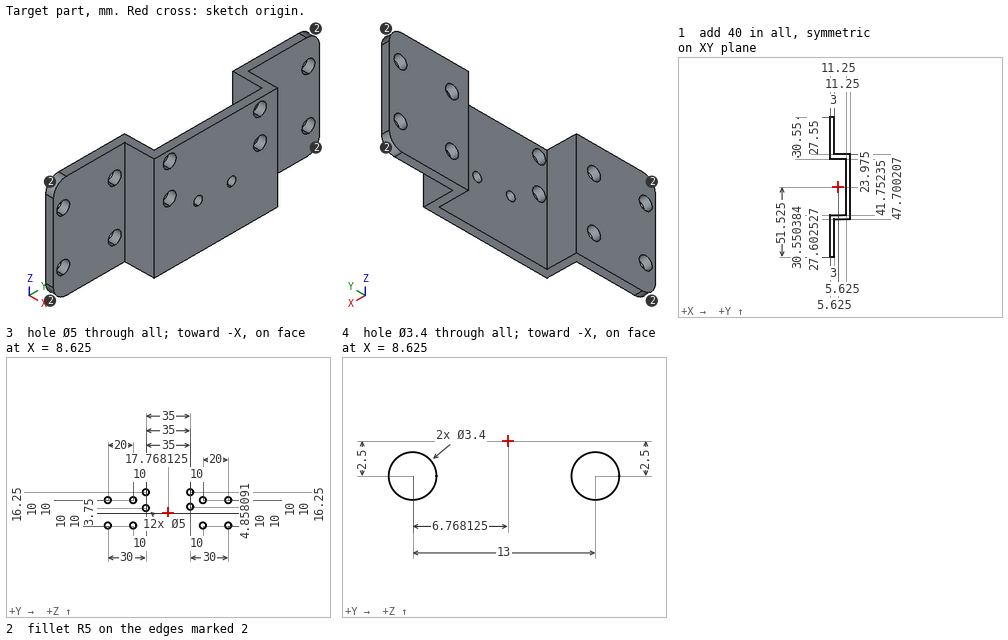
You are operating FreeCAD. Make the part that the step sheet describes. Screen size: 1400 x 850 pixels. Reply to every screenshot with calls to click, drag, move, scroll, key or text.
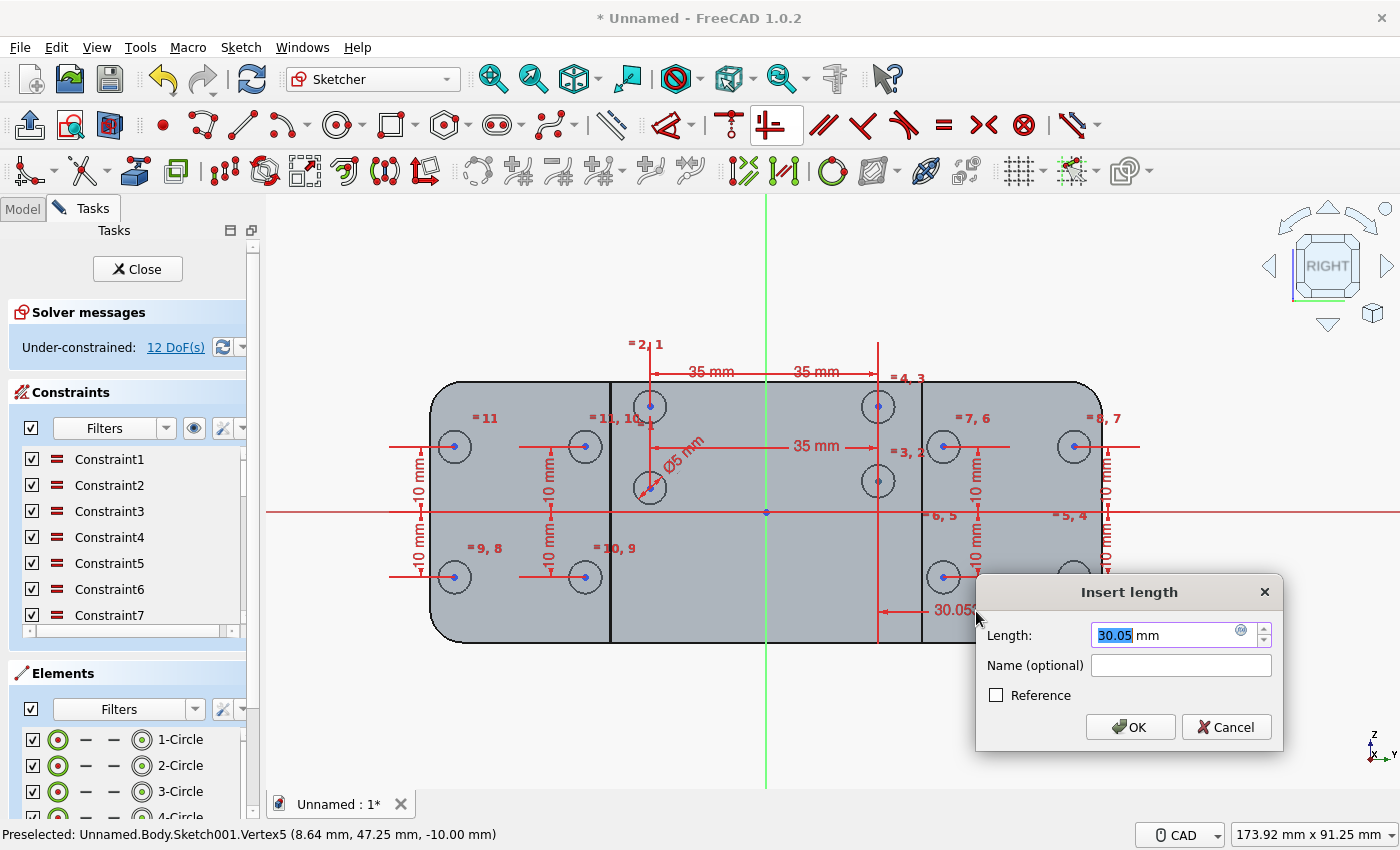
text(30)
key(Return)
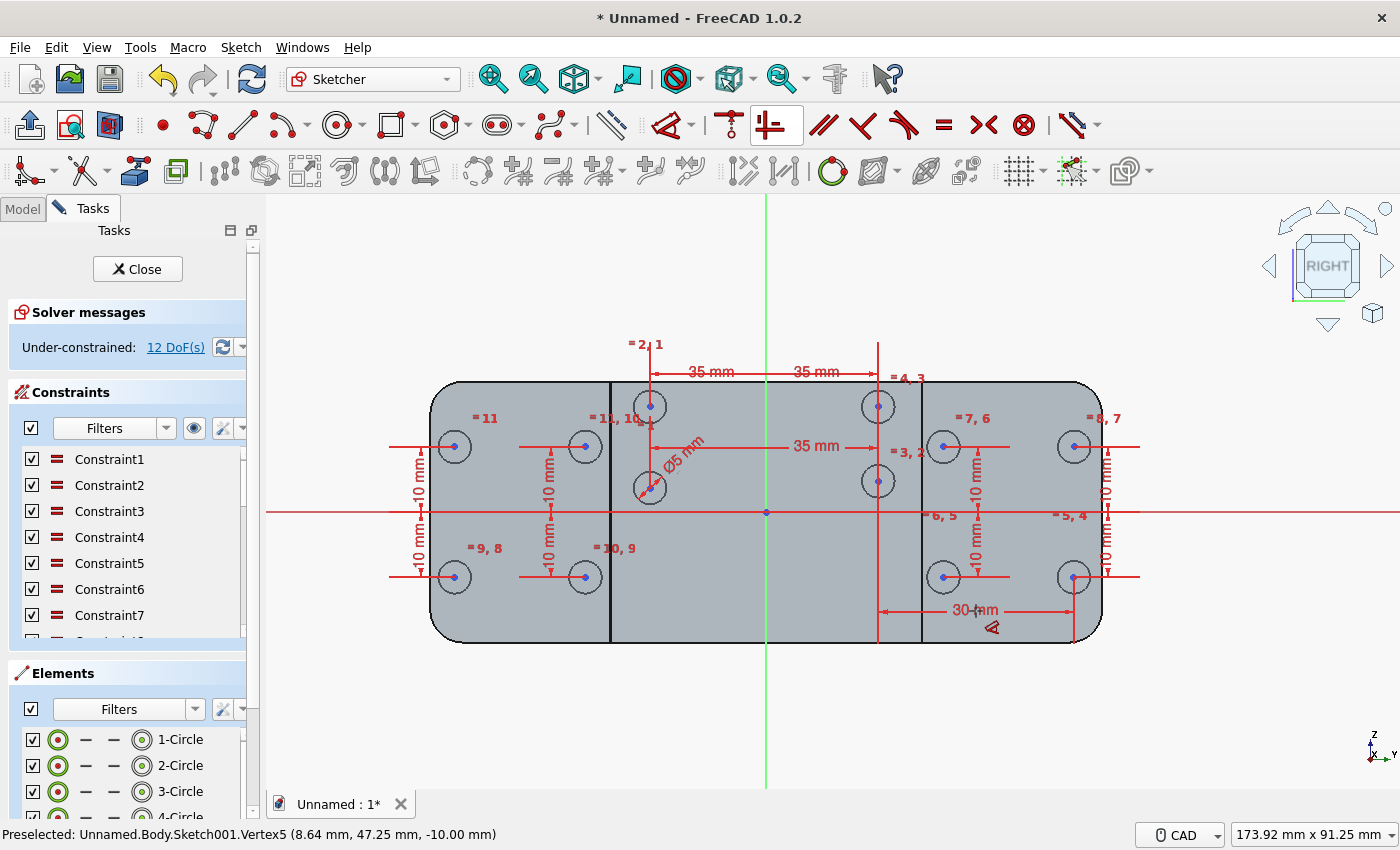
click(878, 481)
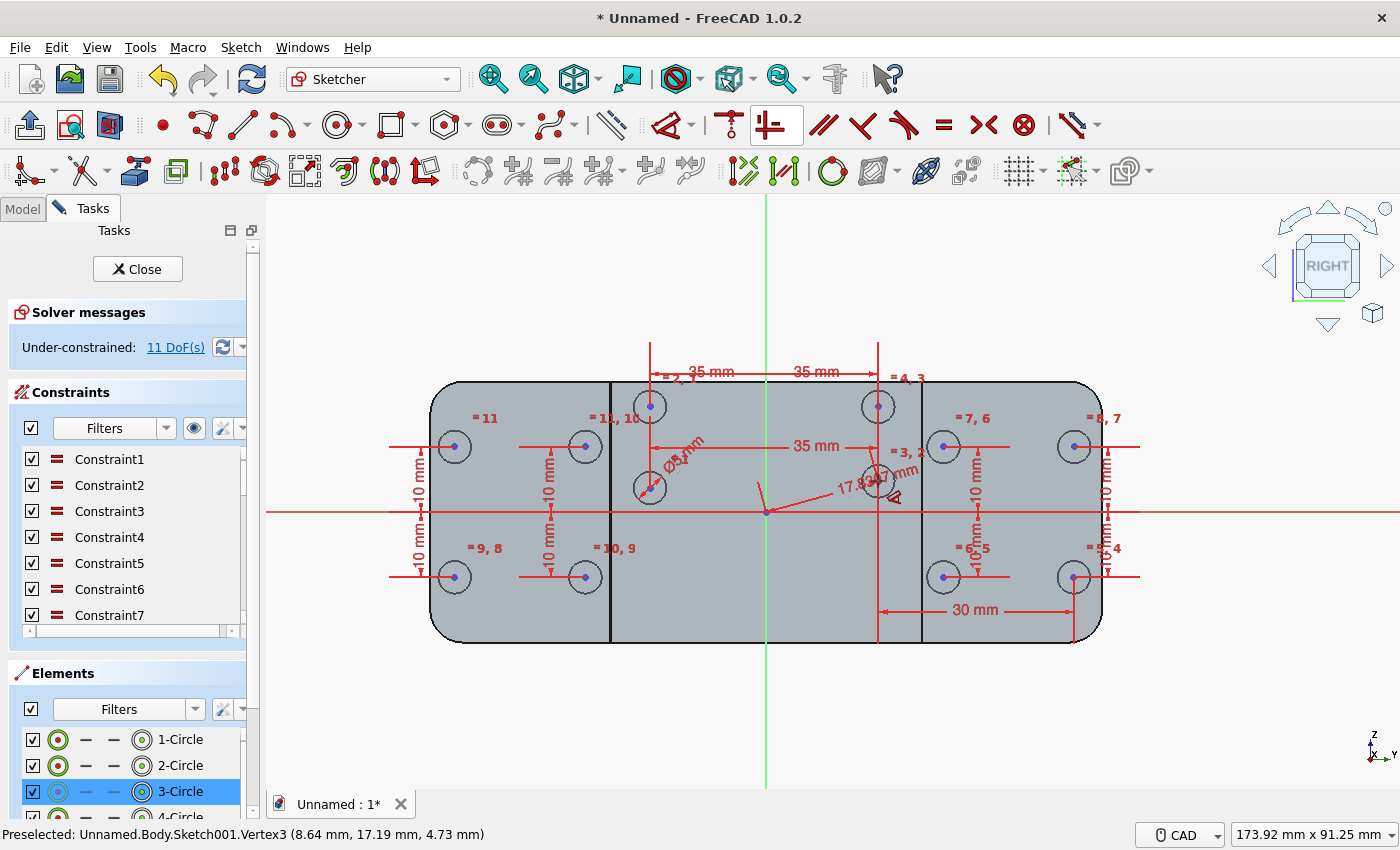
click(944, 577)
click(896, 611)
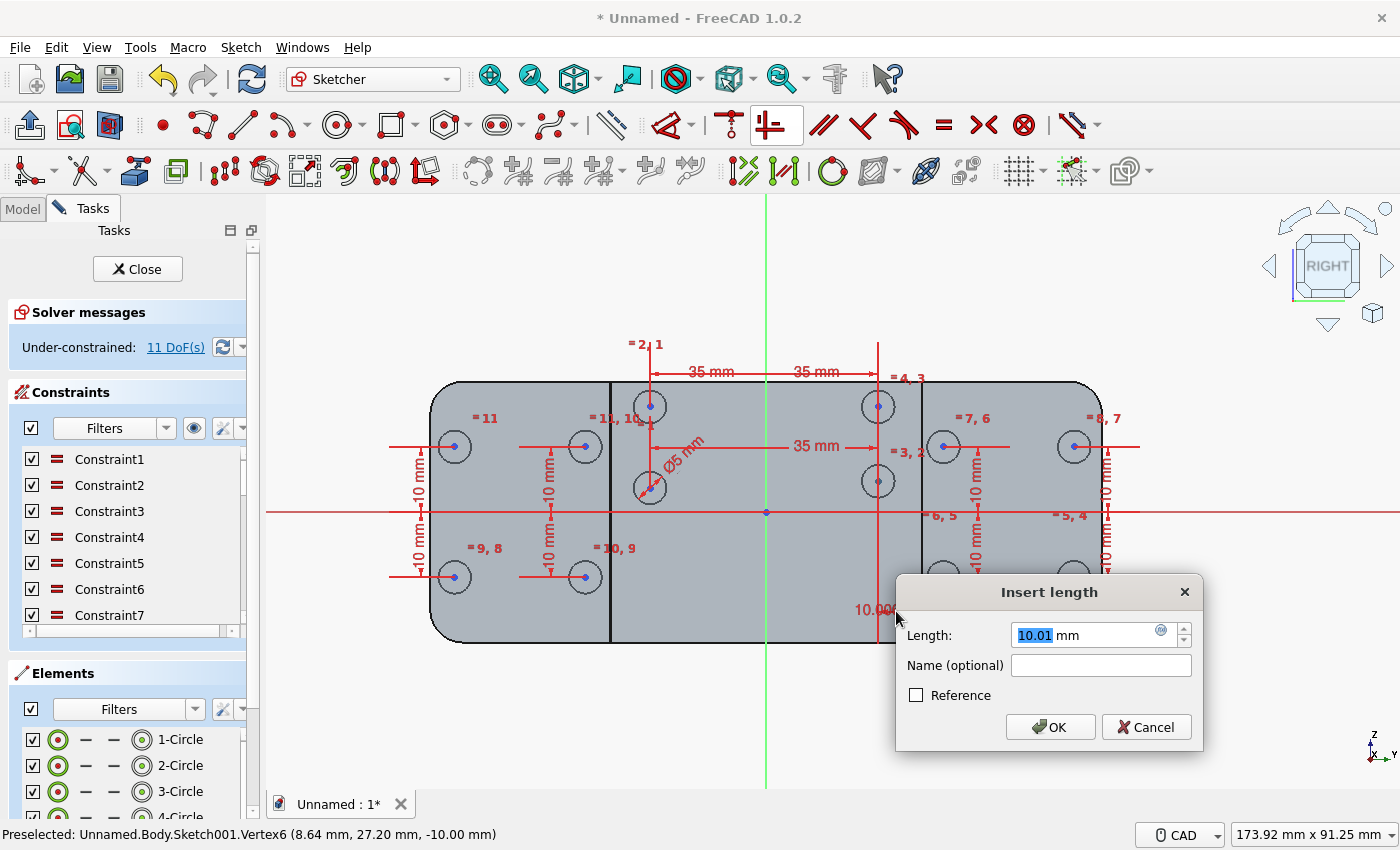
text(10)
key(Return)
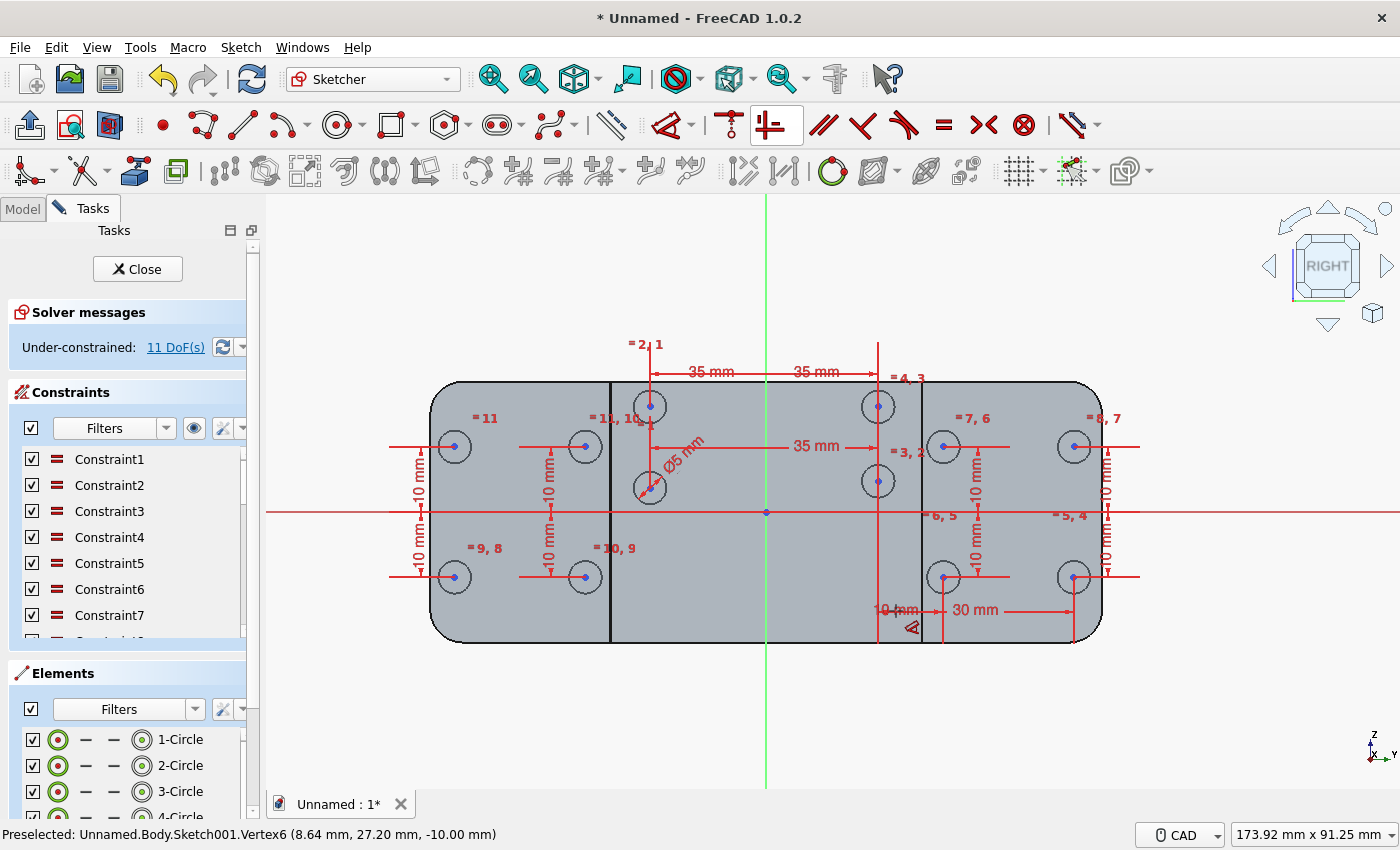
click(878, 481)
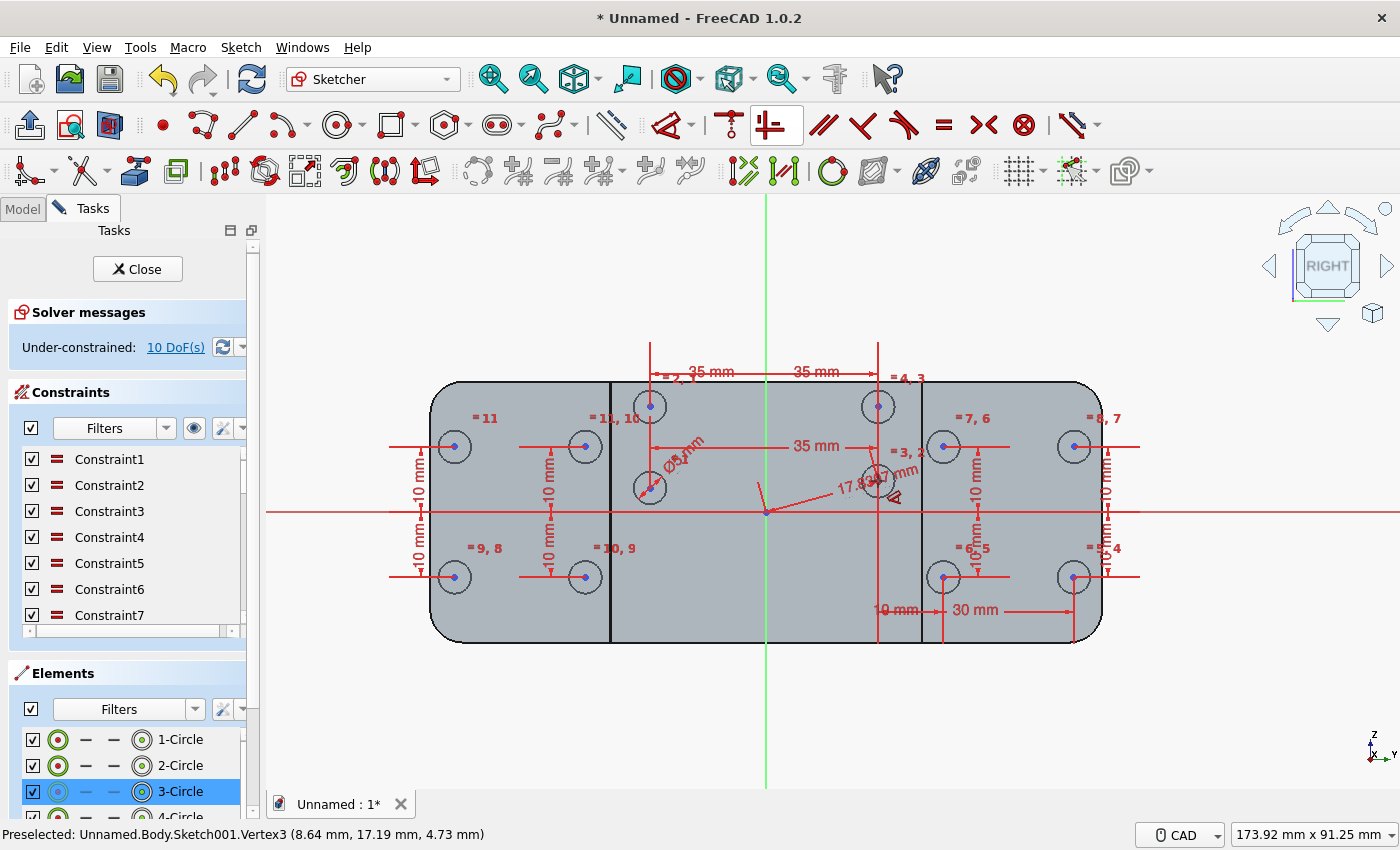
click(944, 447)
click(911, 413)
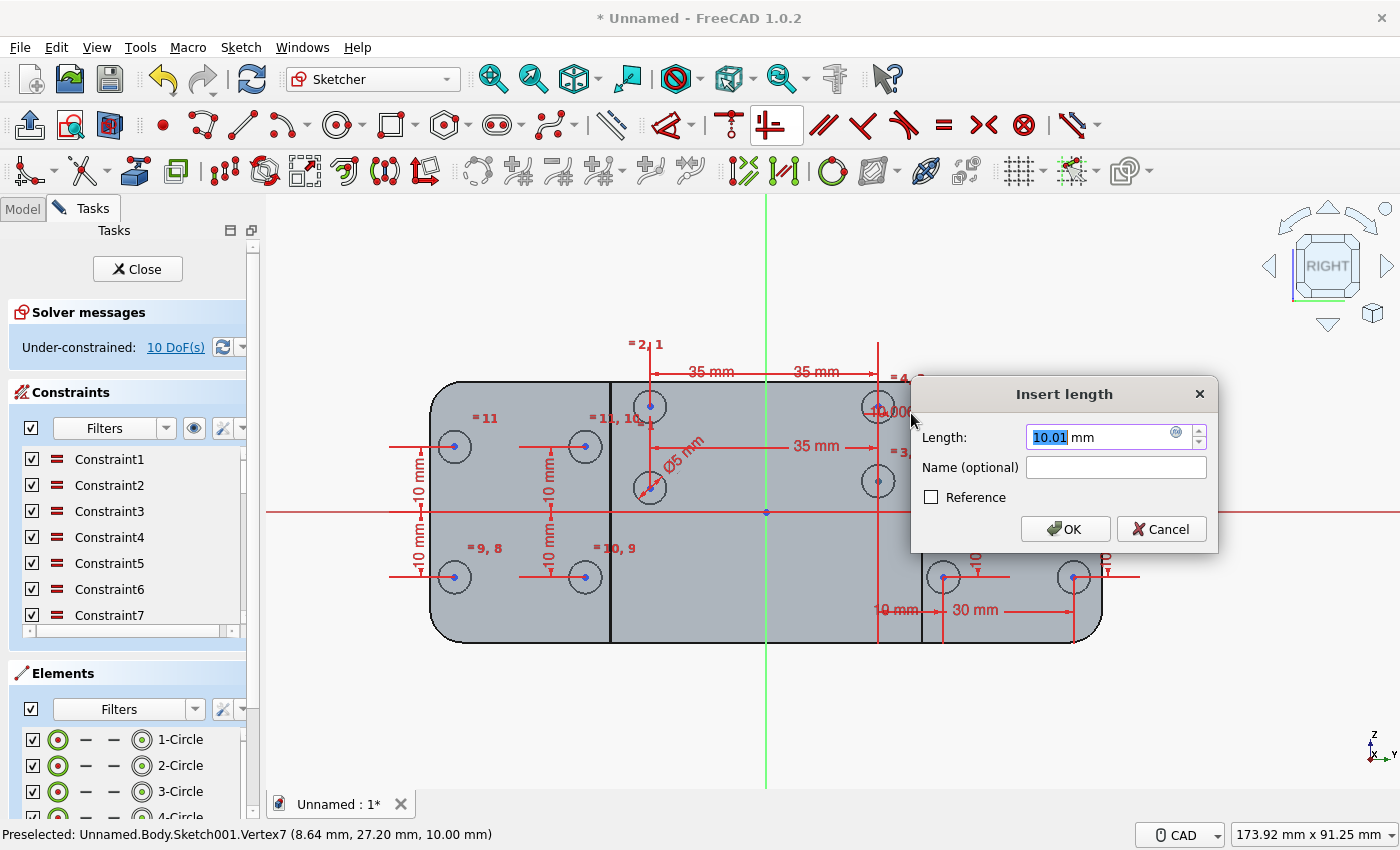
text(10)
key(Return)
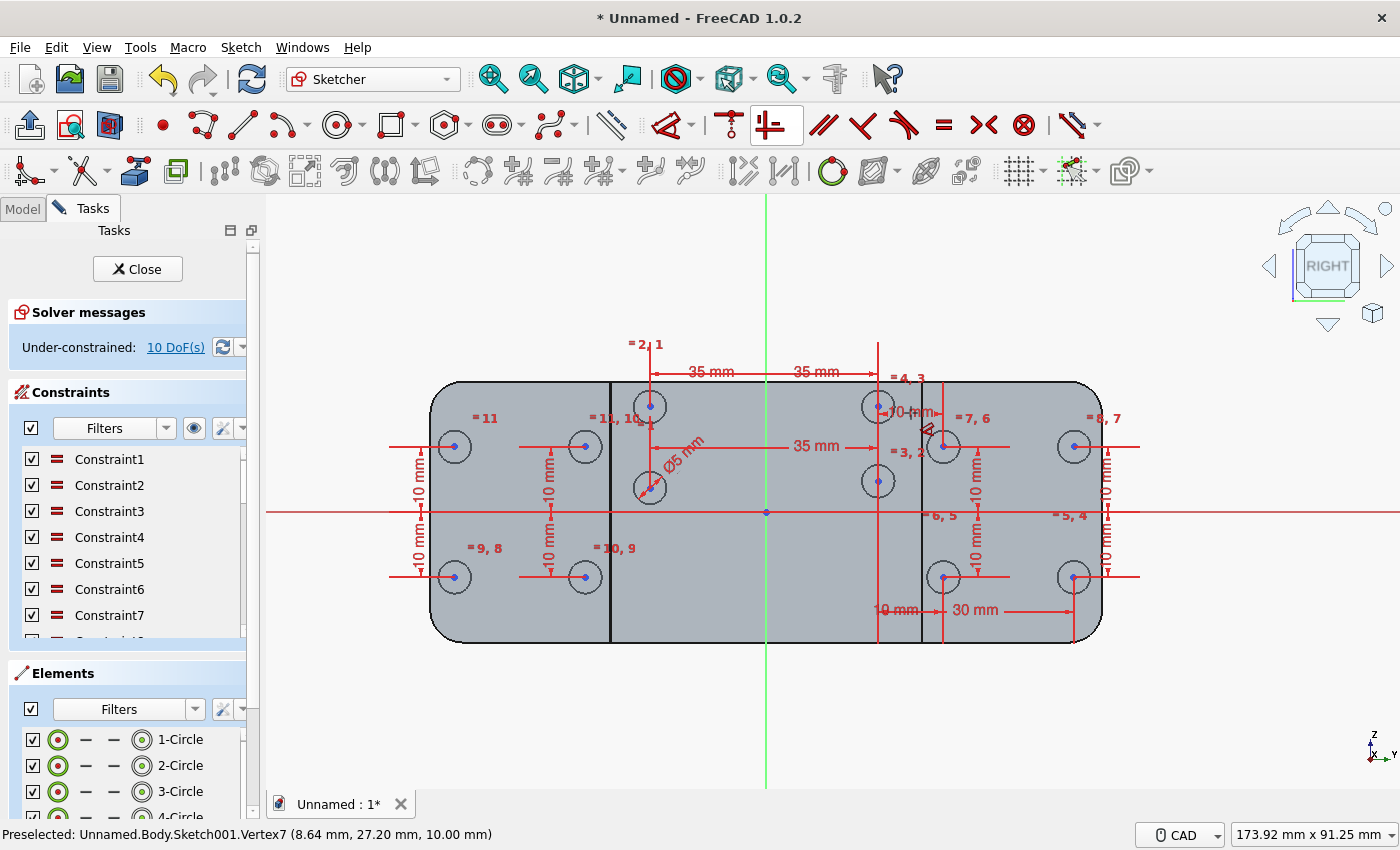
click(943, 447)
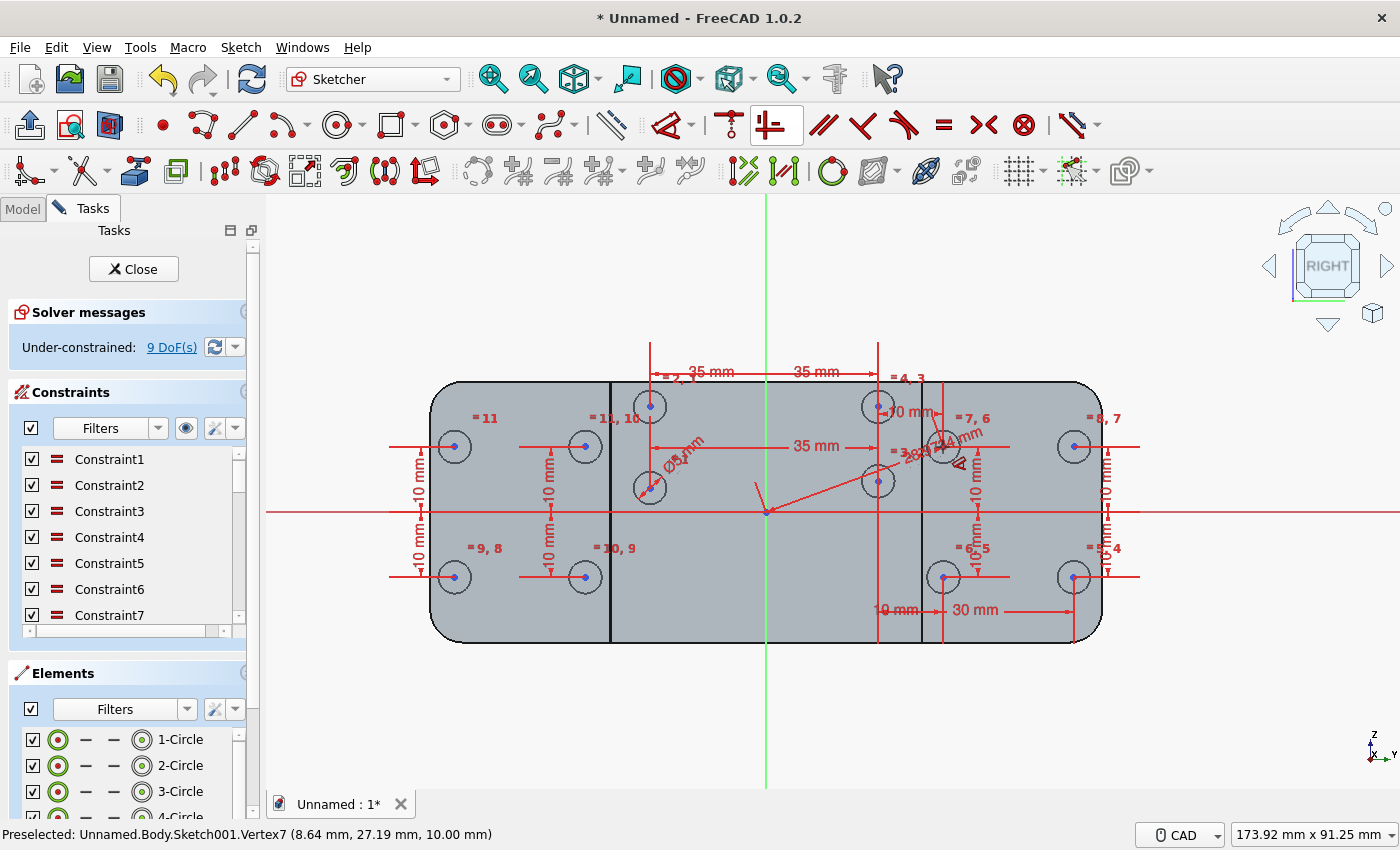
click(1074, 447)
click(1009, 413)